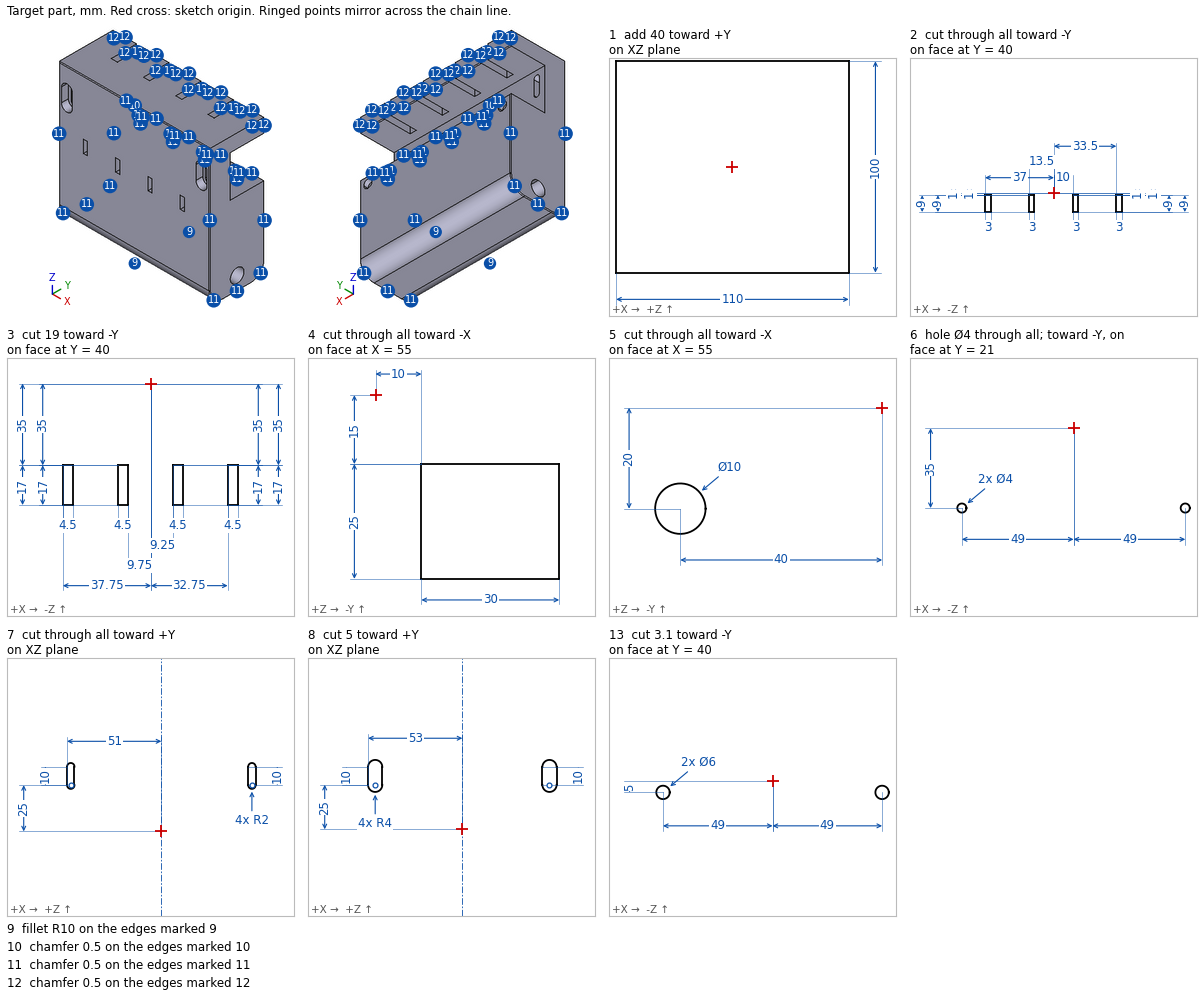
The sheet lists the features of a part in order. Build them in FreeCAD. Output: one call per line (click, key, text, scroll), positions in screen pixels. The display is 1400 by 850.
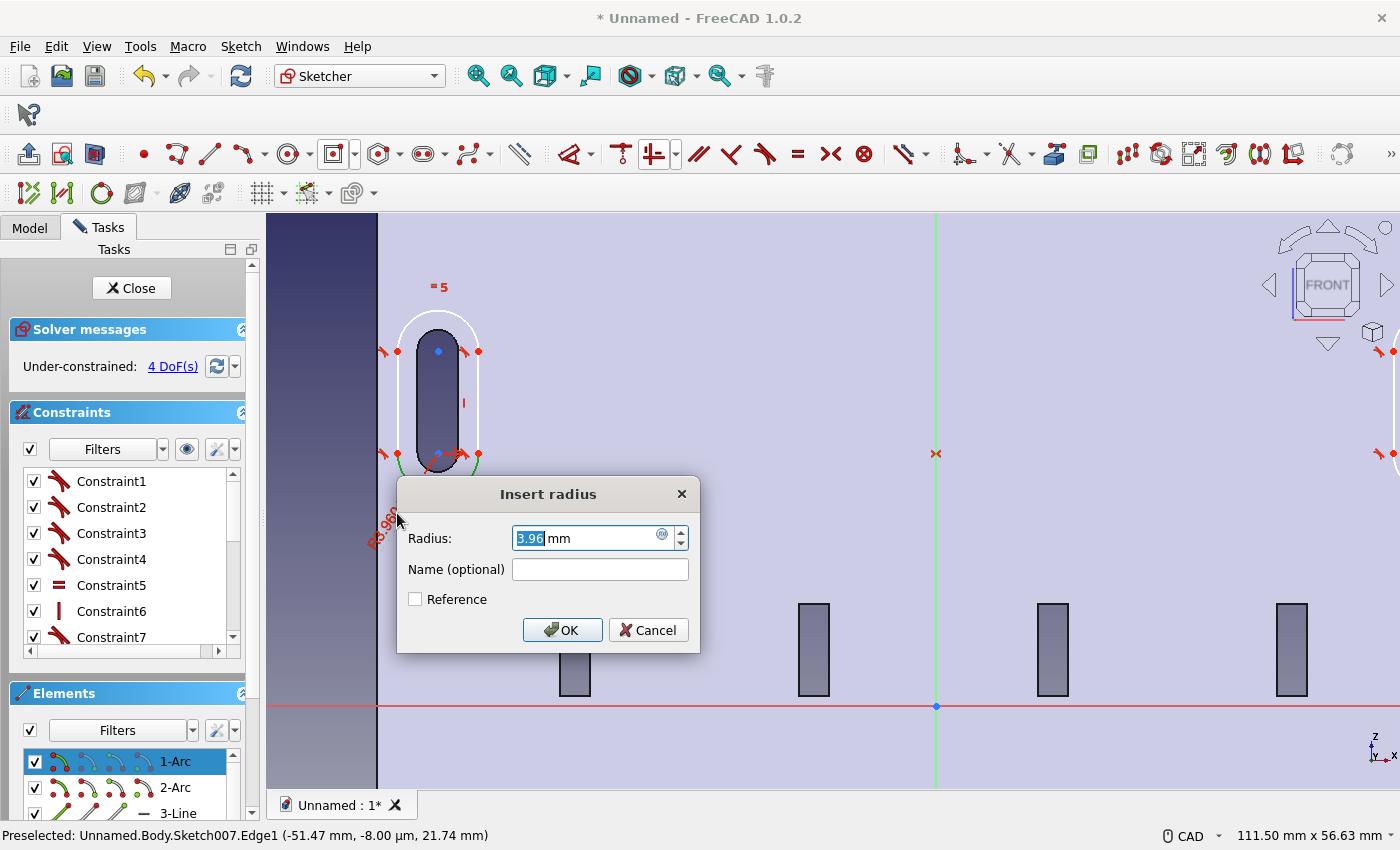
text(4)
key(Return)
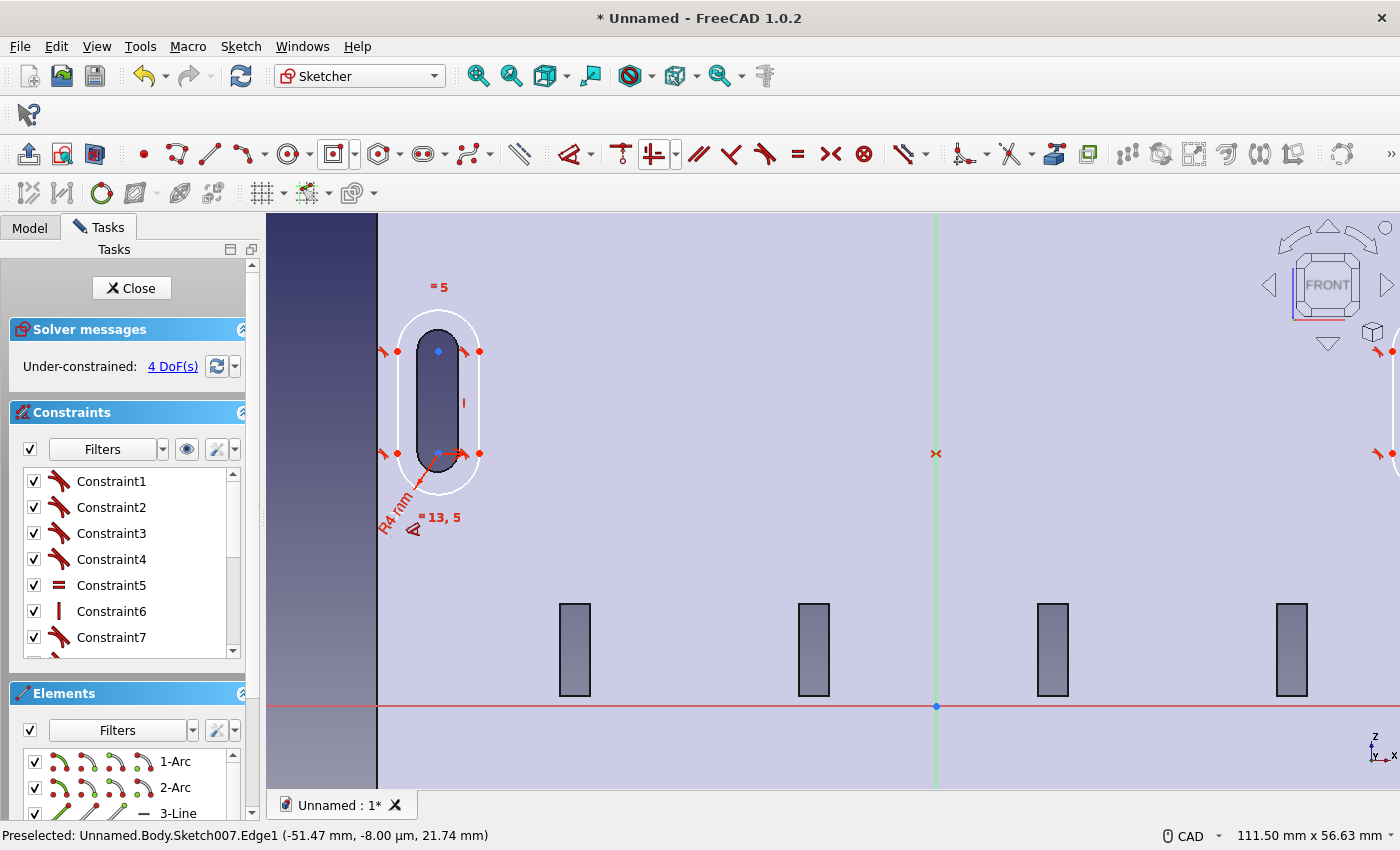
click(398, 423)
click(364, 402)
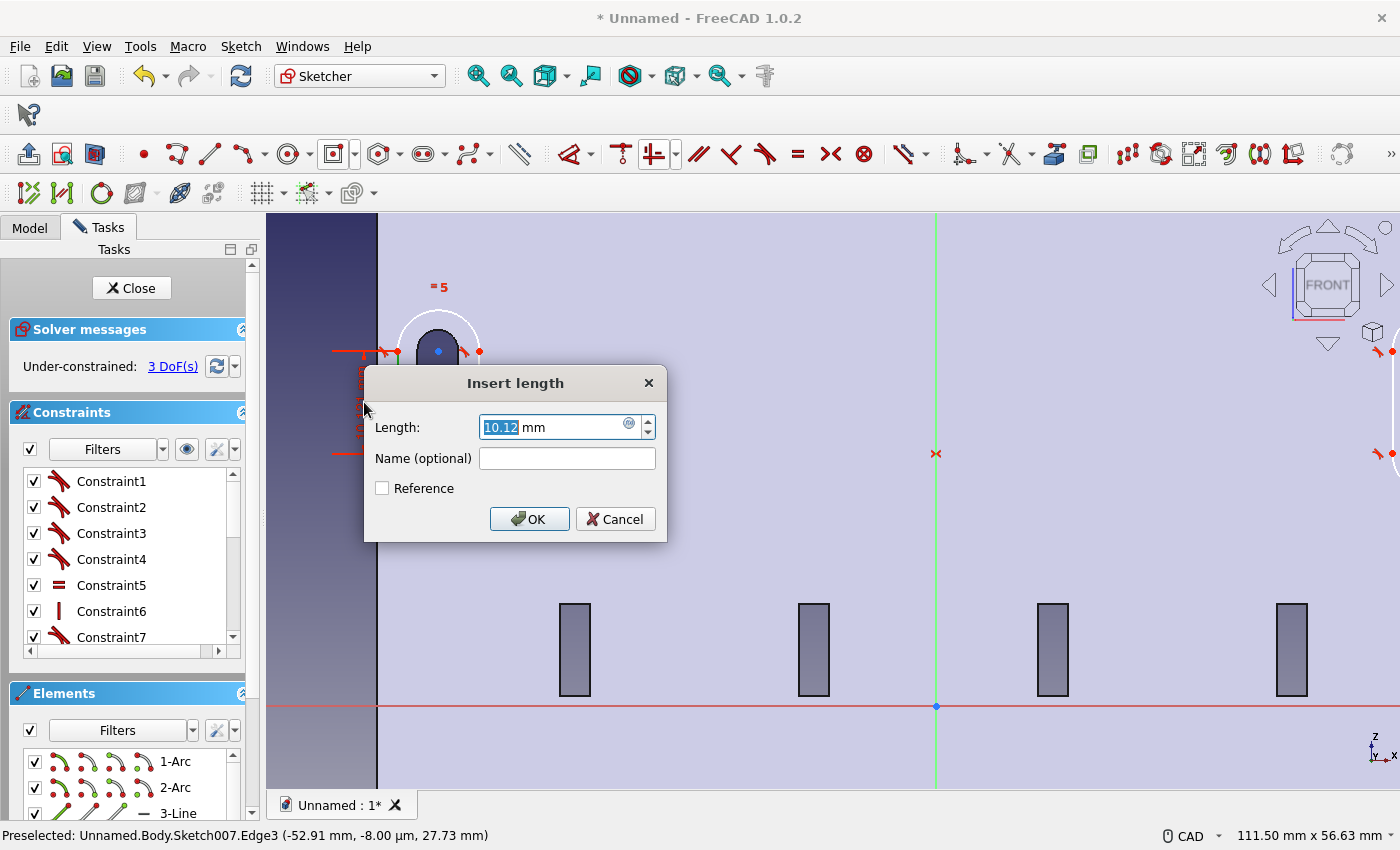
text(10)
key(Return)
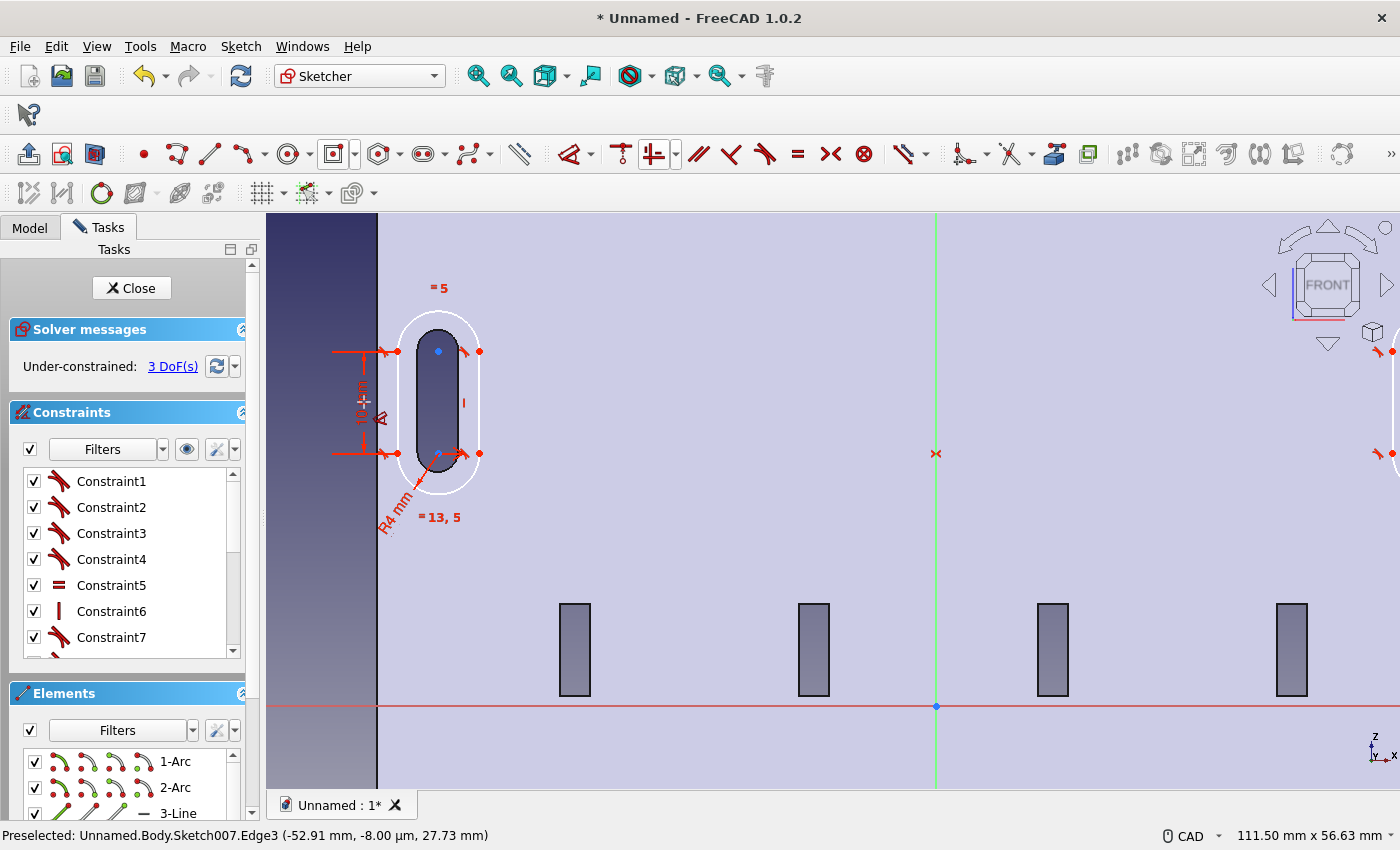
scroll(416, 487, down, 2)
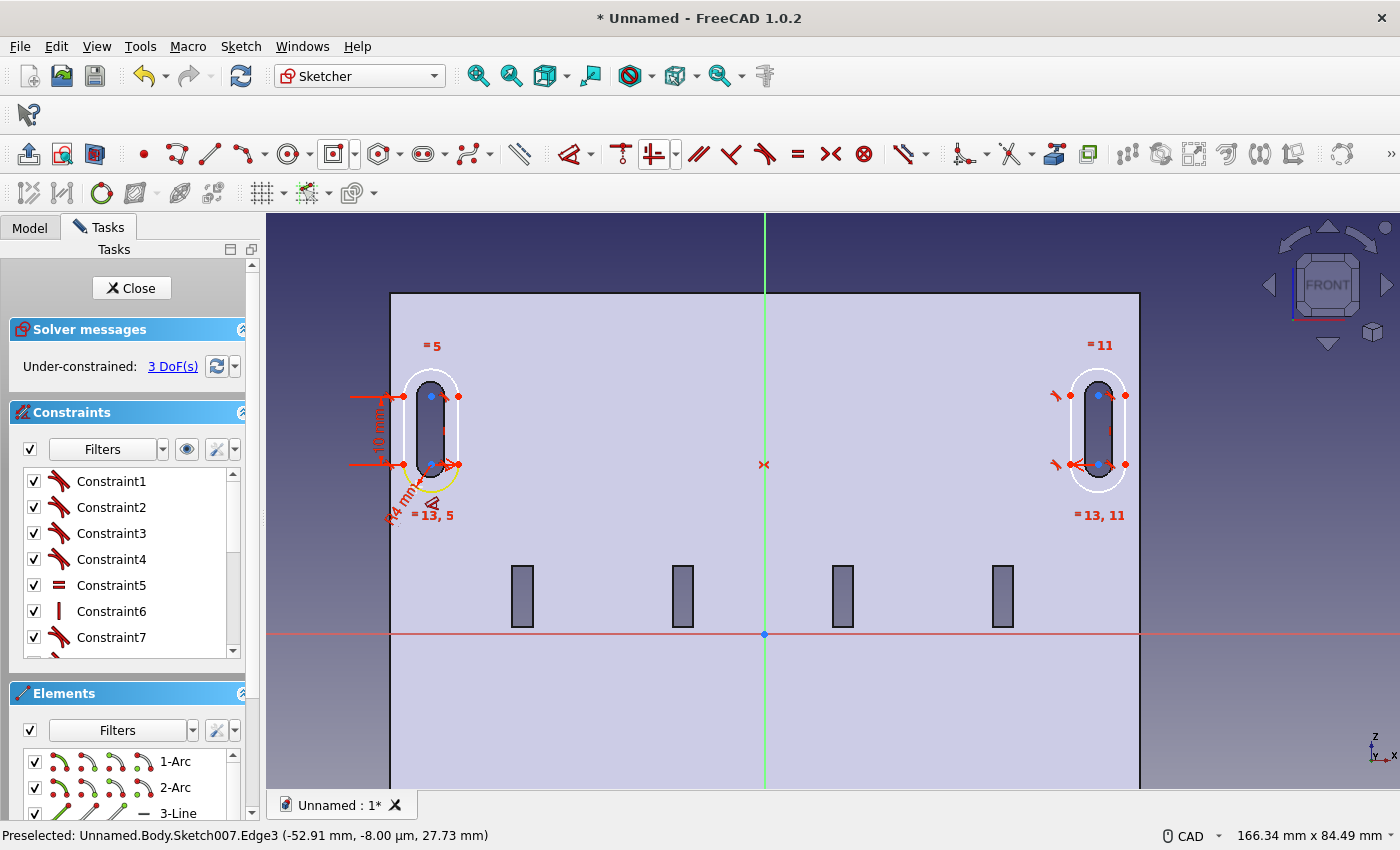
click(1071, 444)
click(1105, 430)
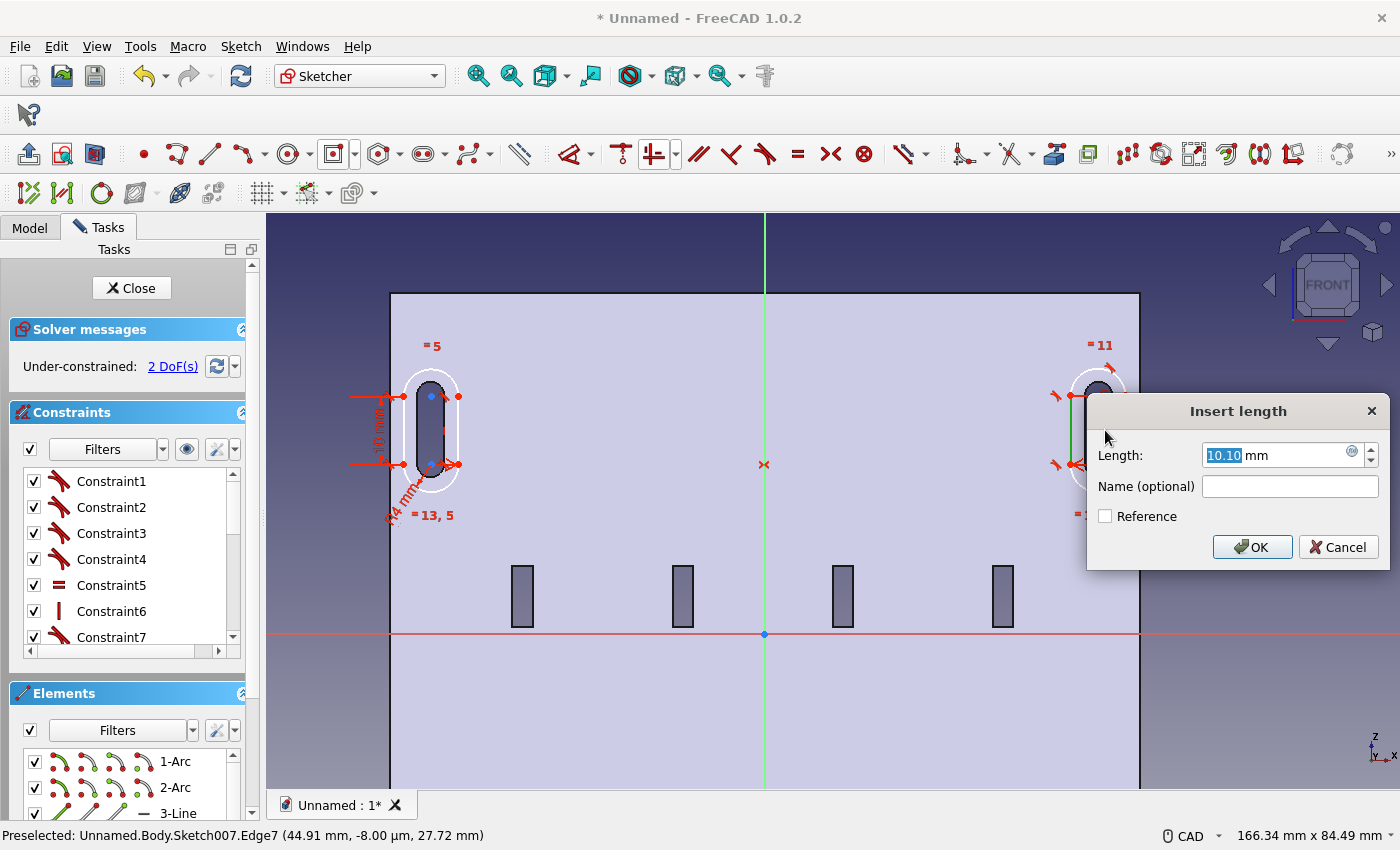
text(10)
key(Return)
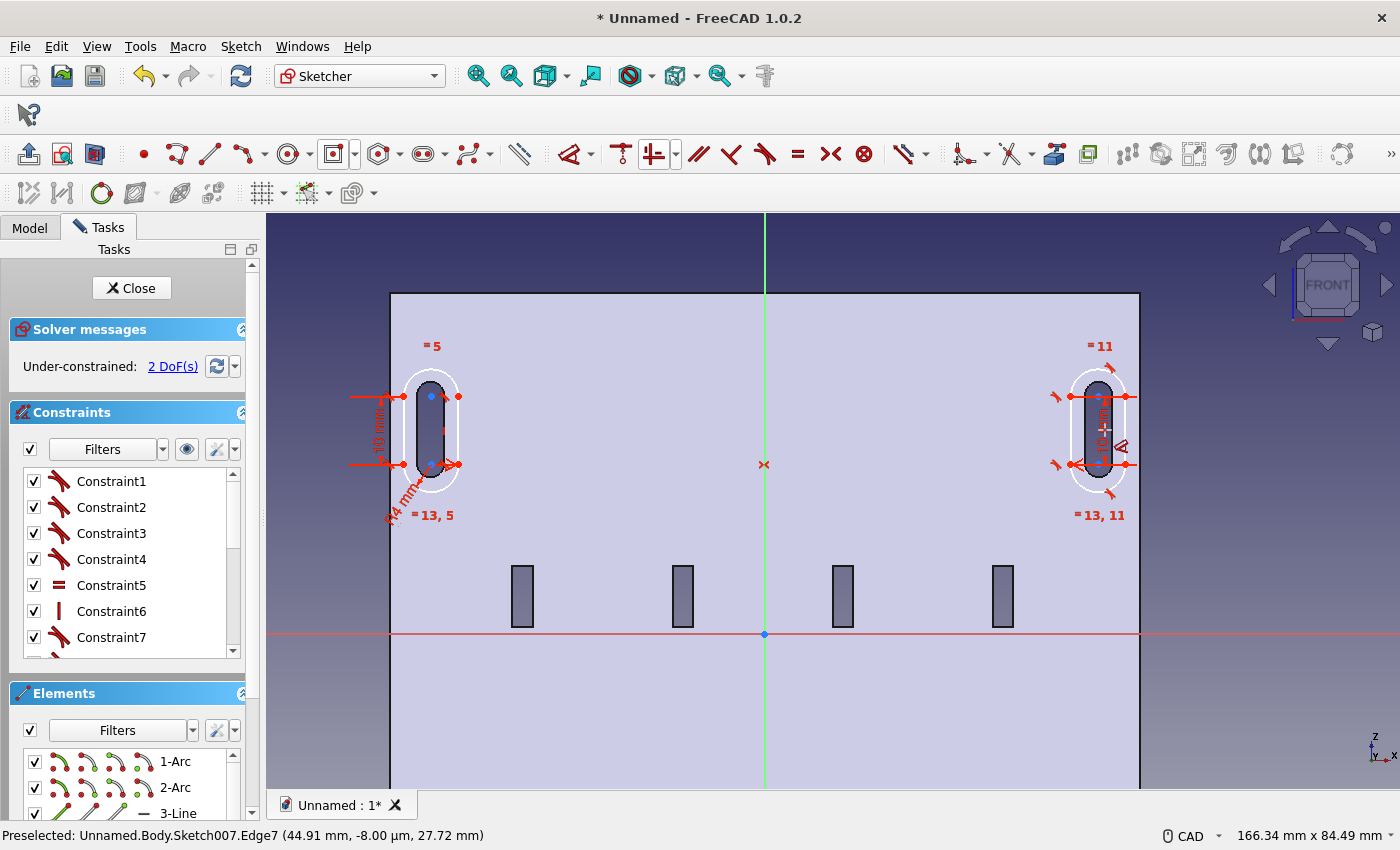
click(404, 465)
click(584, 668)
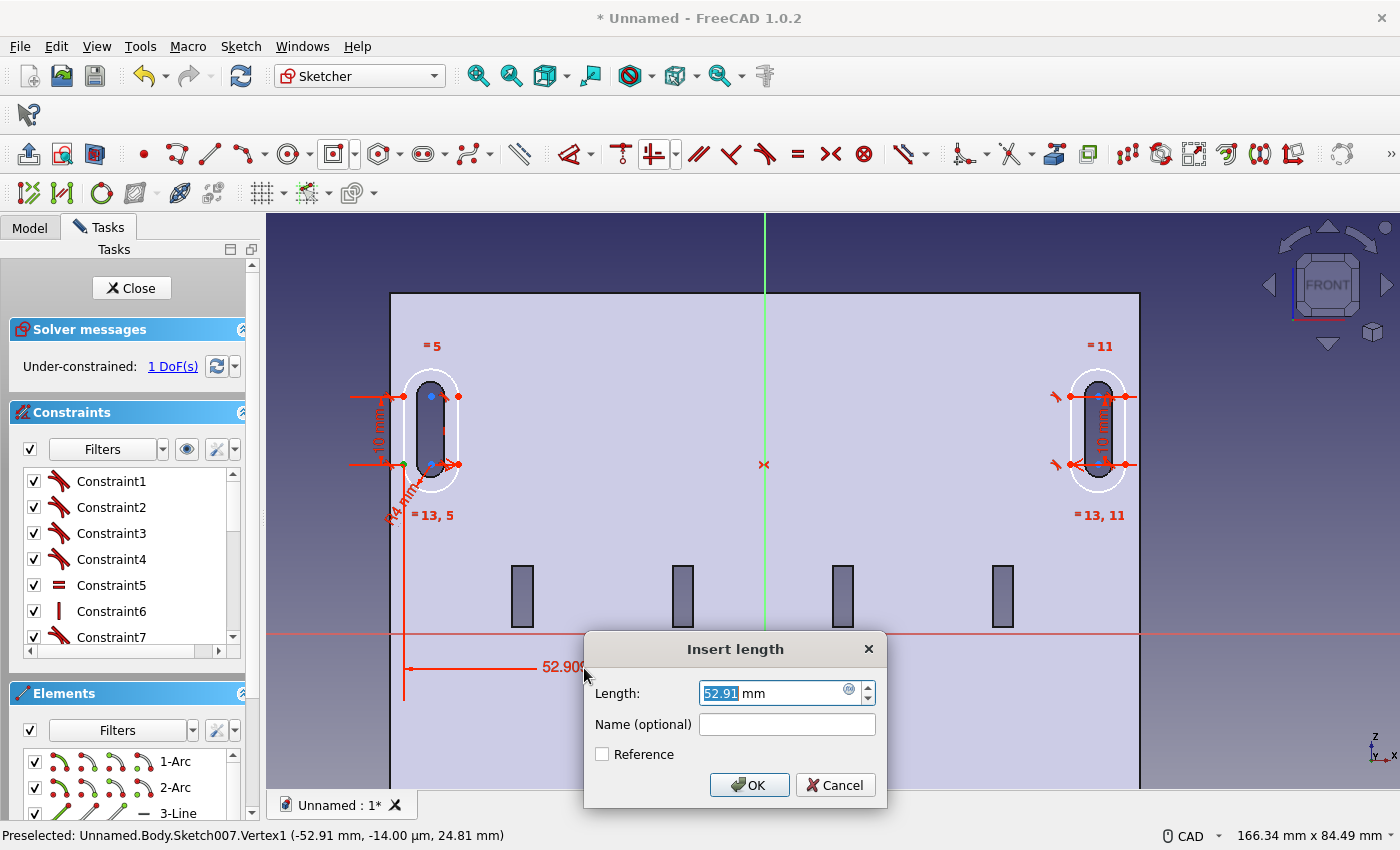
text(53)
key(Return)